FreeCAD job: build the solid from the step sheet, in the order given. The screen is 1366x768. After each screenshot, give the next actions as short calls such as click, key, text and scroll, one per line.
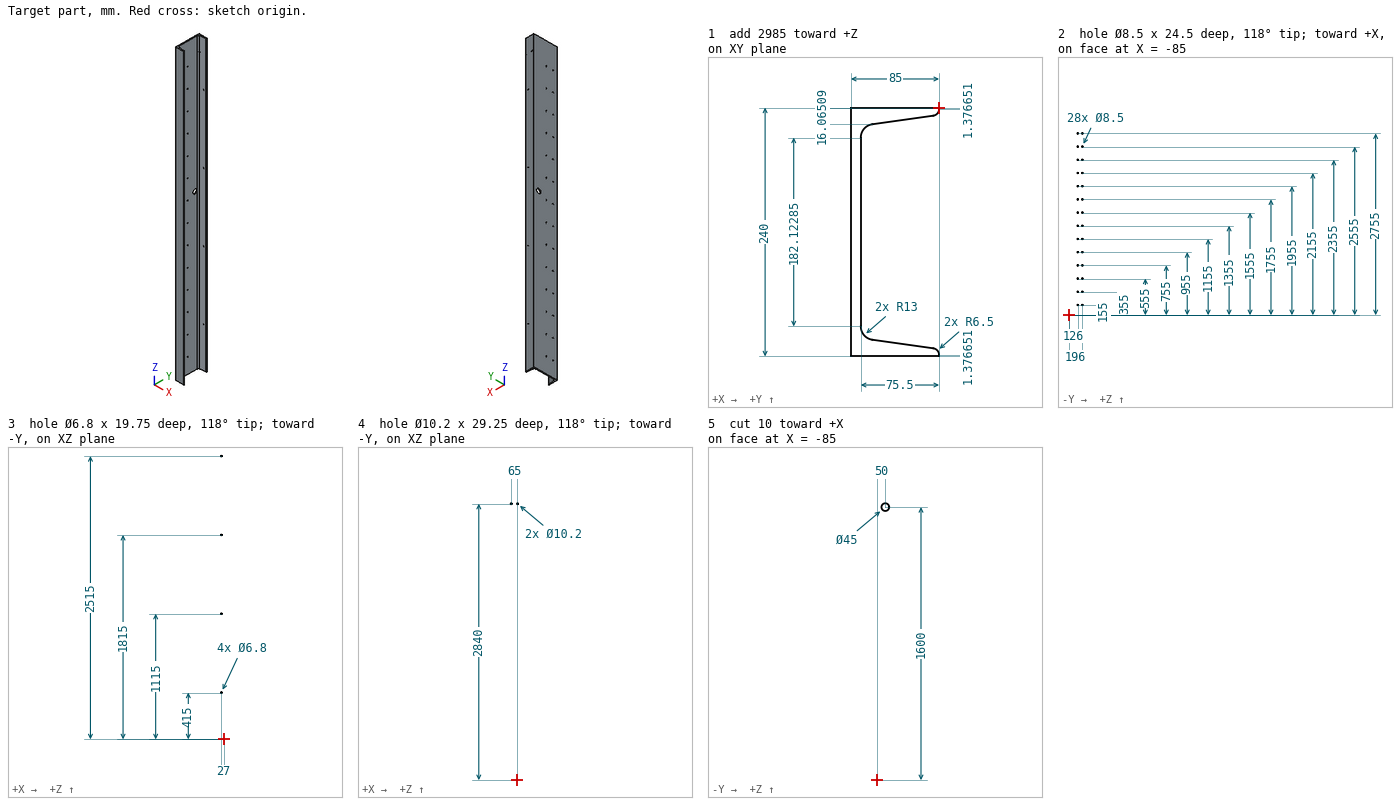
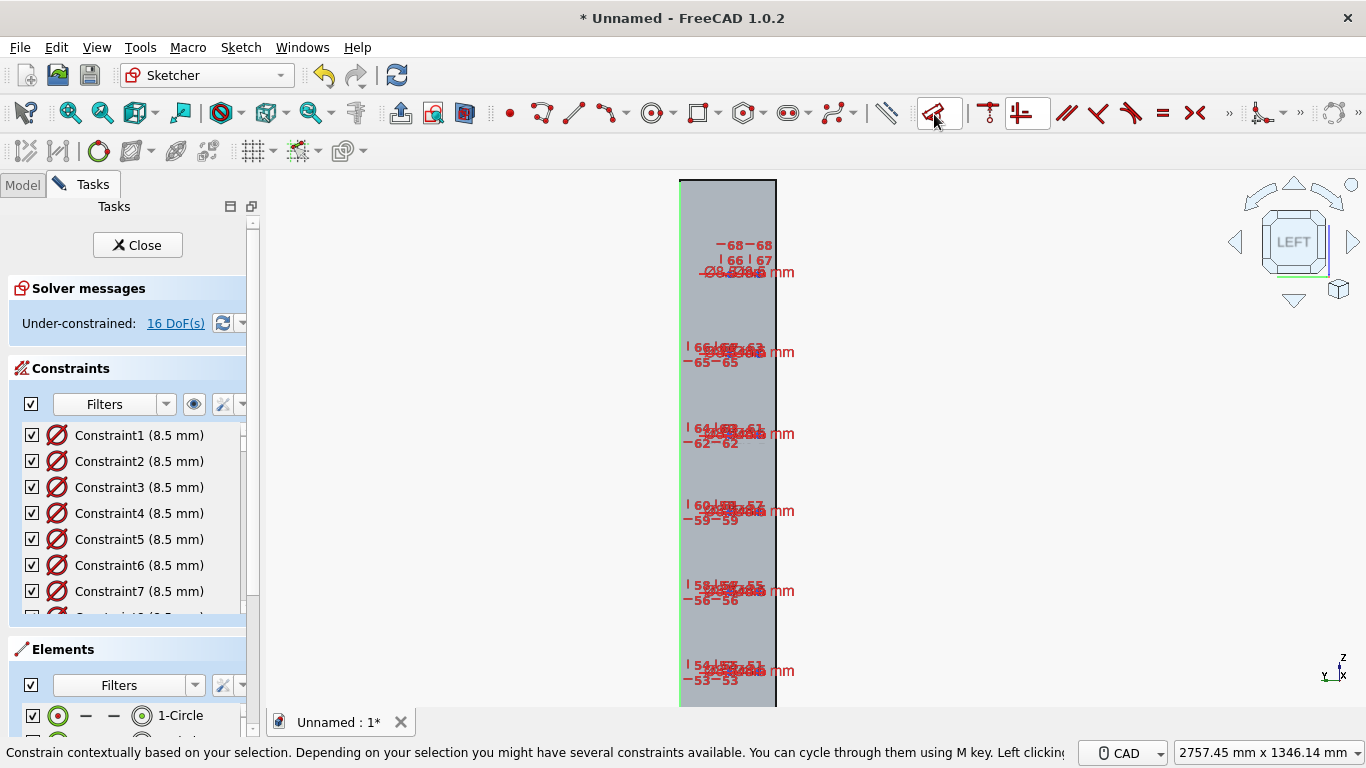
scroll(759, 274, down, 6)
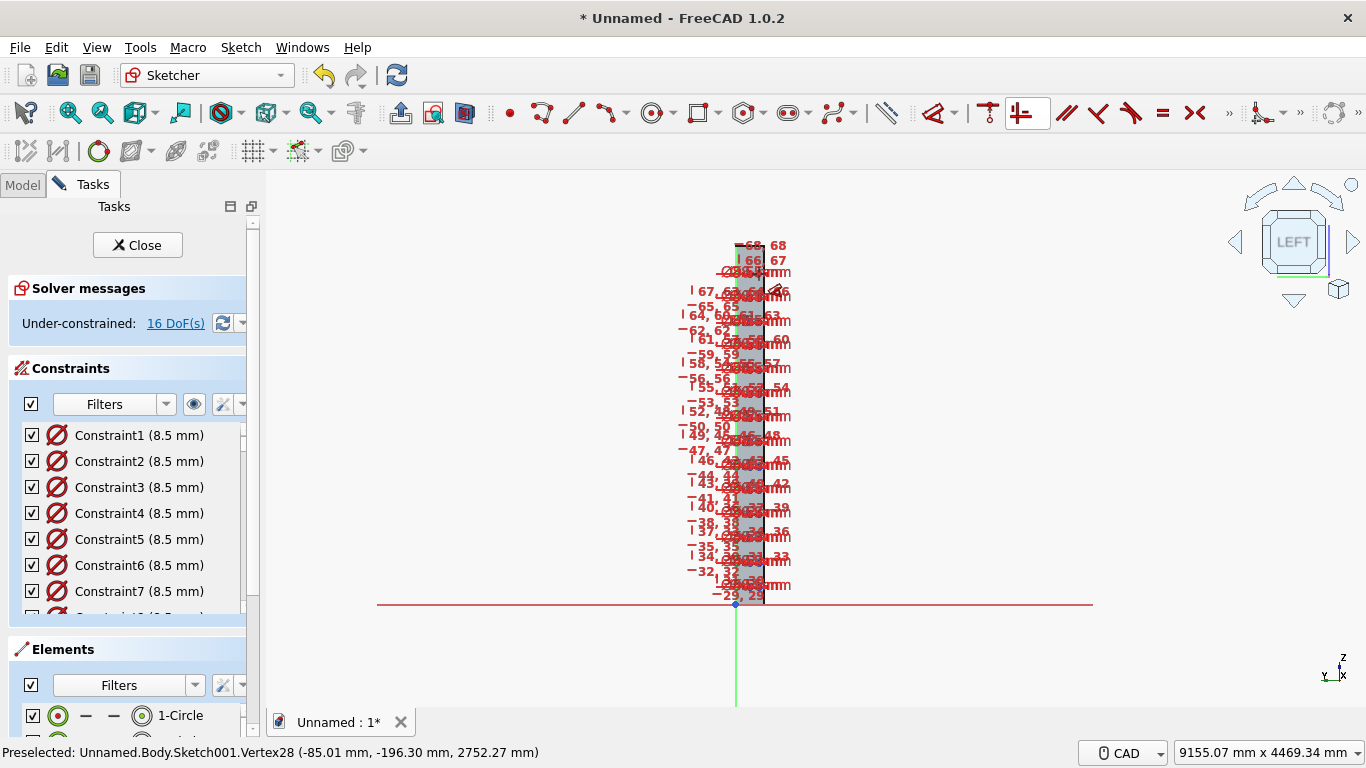
scroll(750, 587, up, 5)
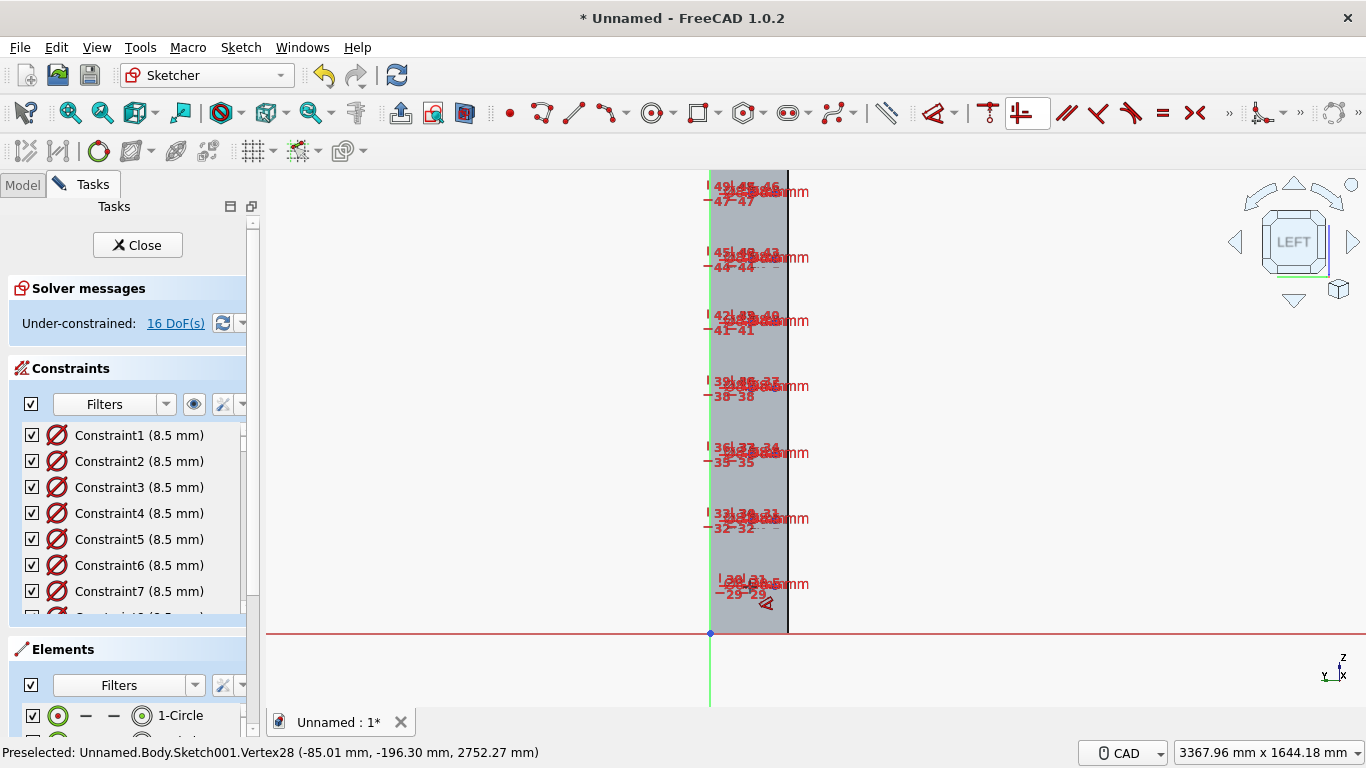
click(750, 586)
click(730, 668)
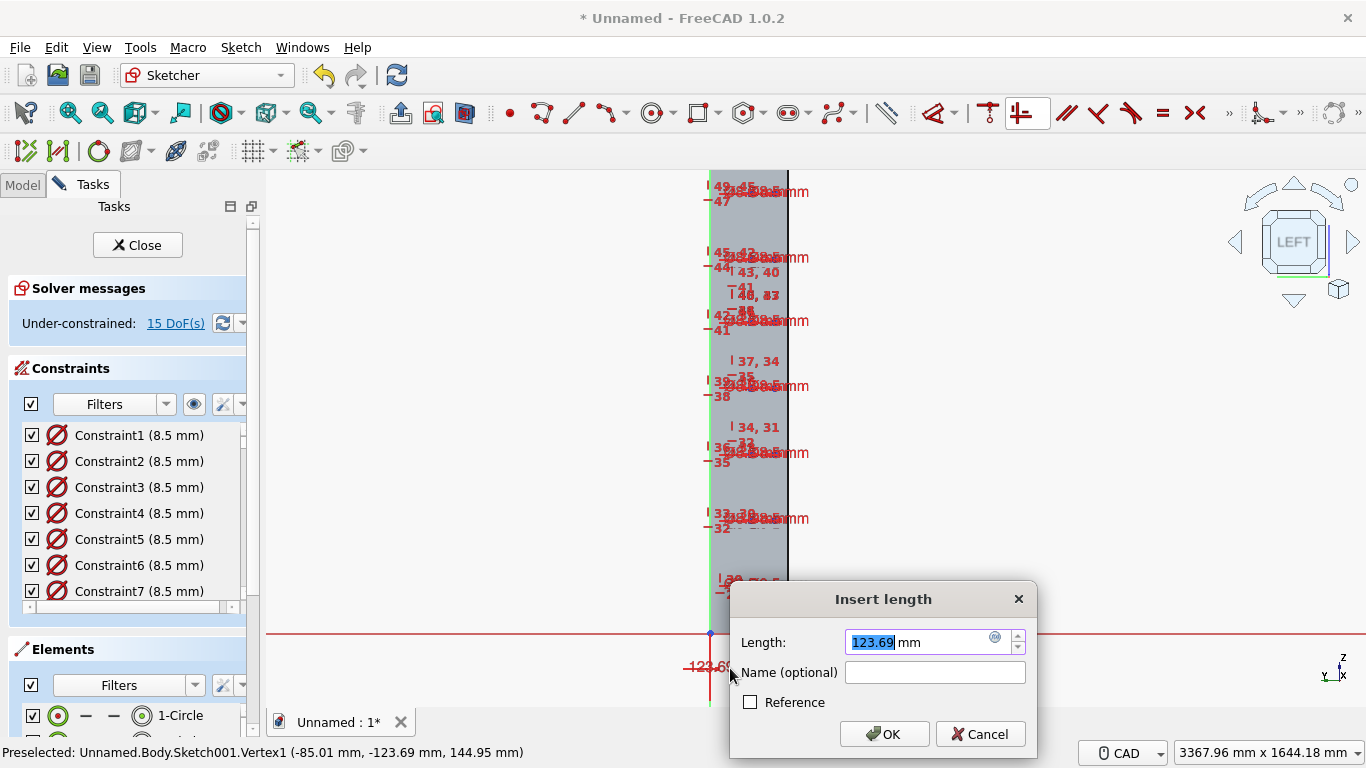
text(126)
key(Return)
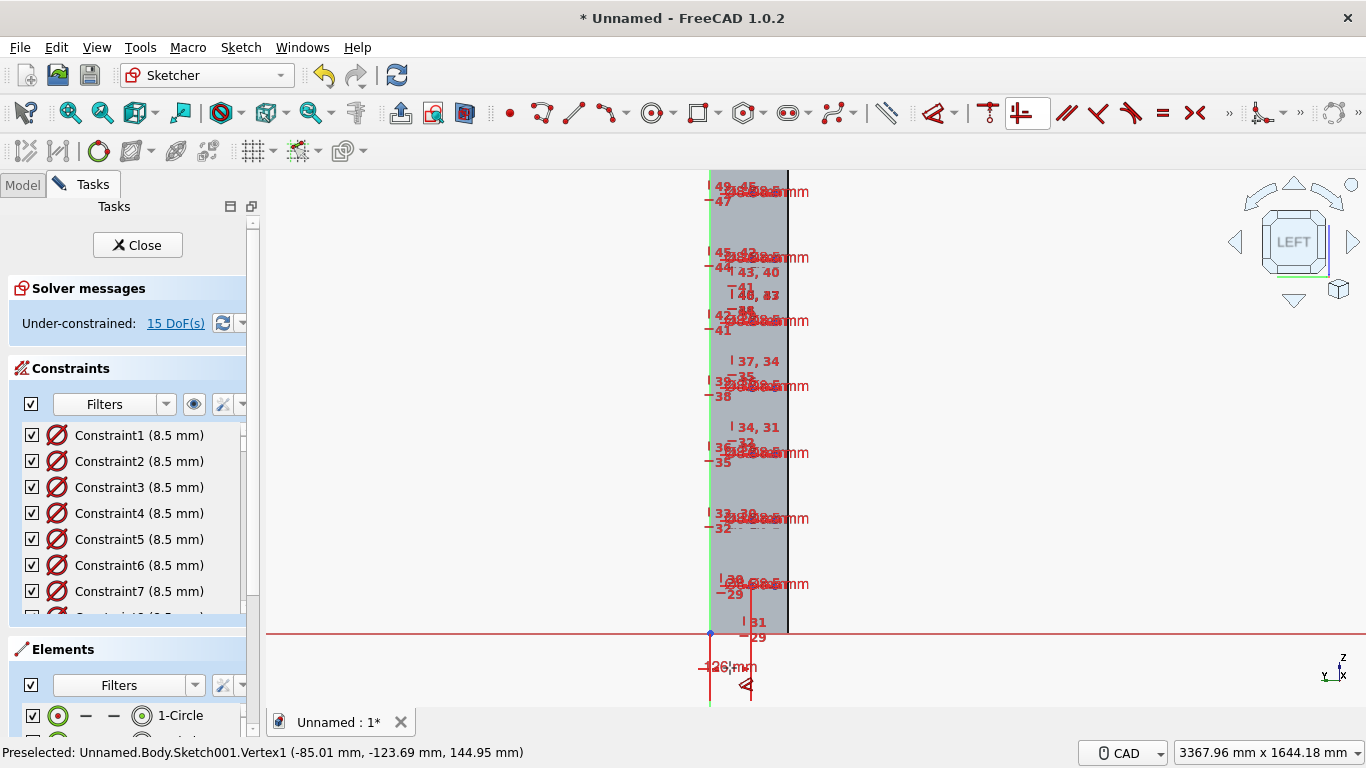
click(751, 586)
click(676, 610)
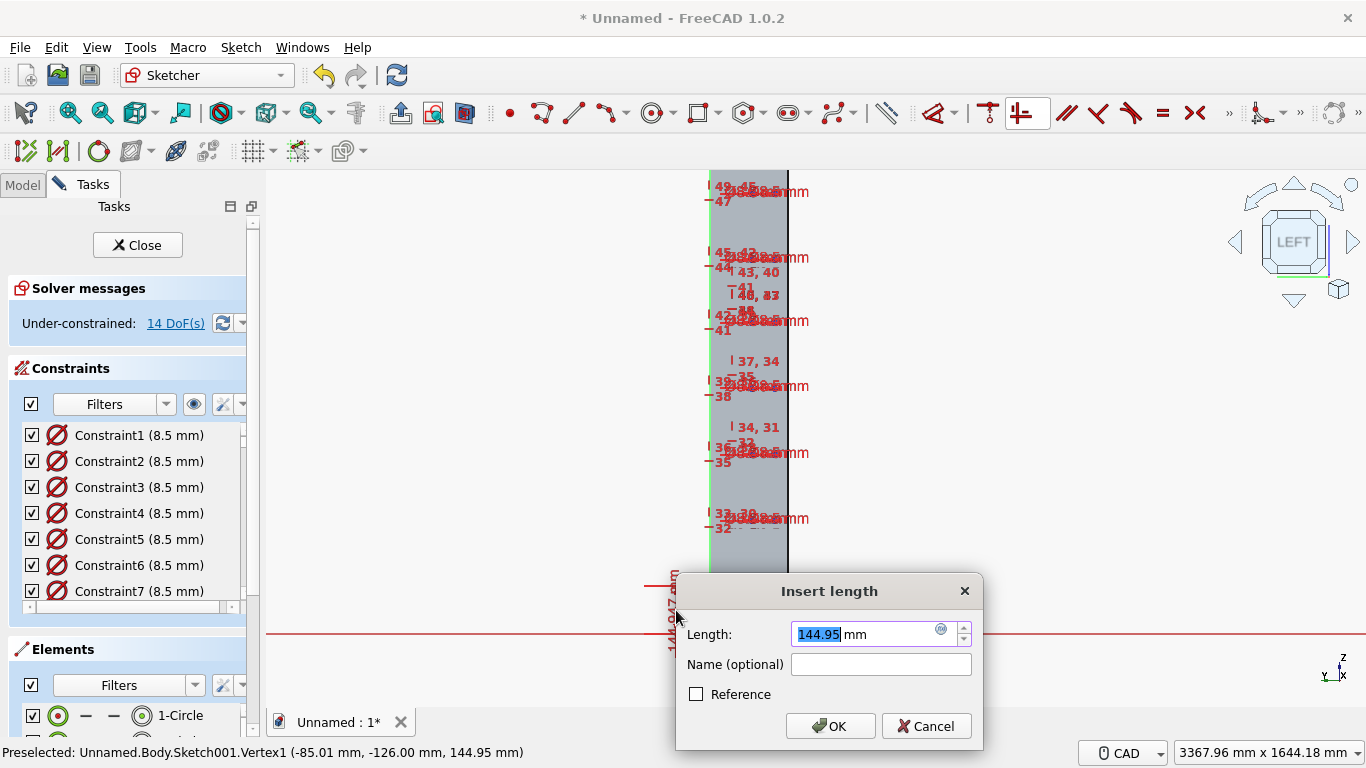
text(155)
key(Return)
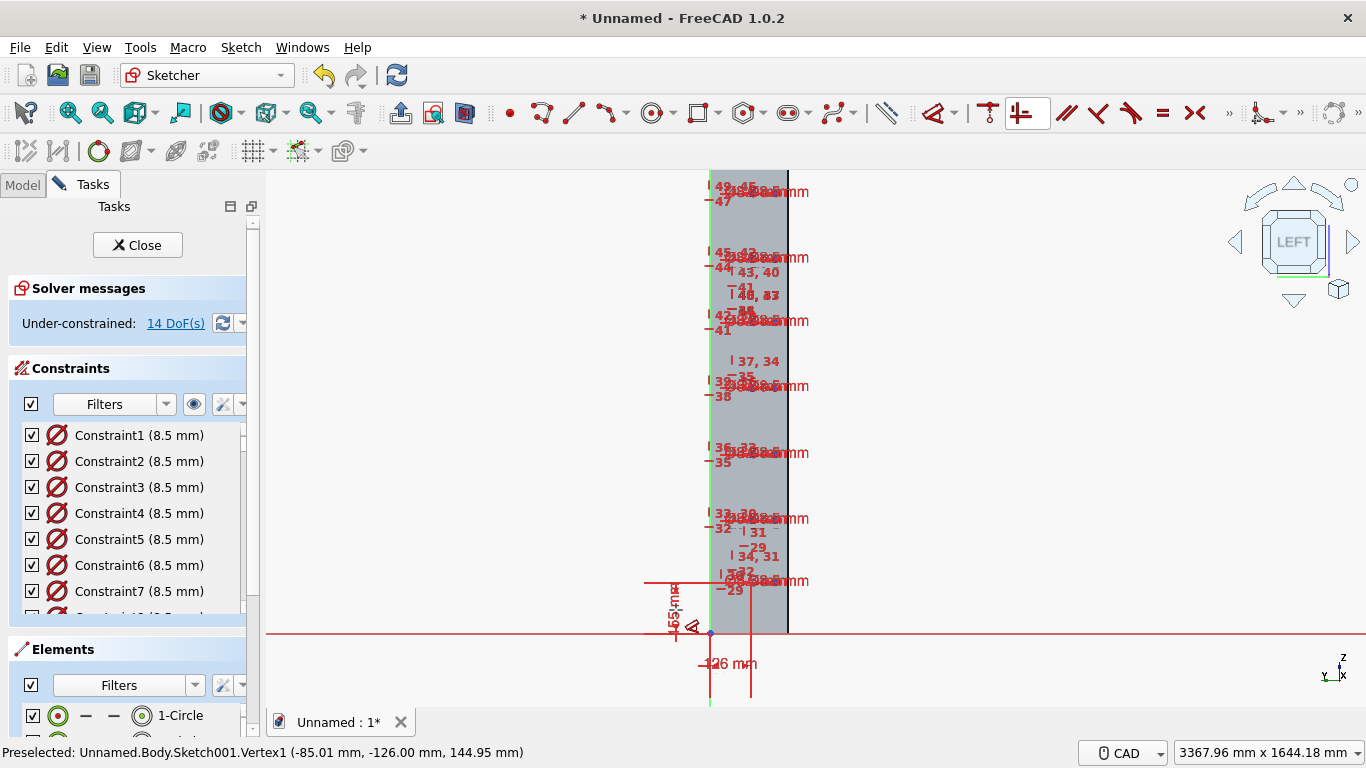
click(774, 583)
click(742, 549)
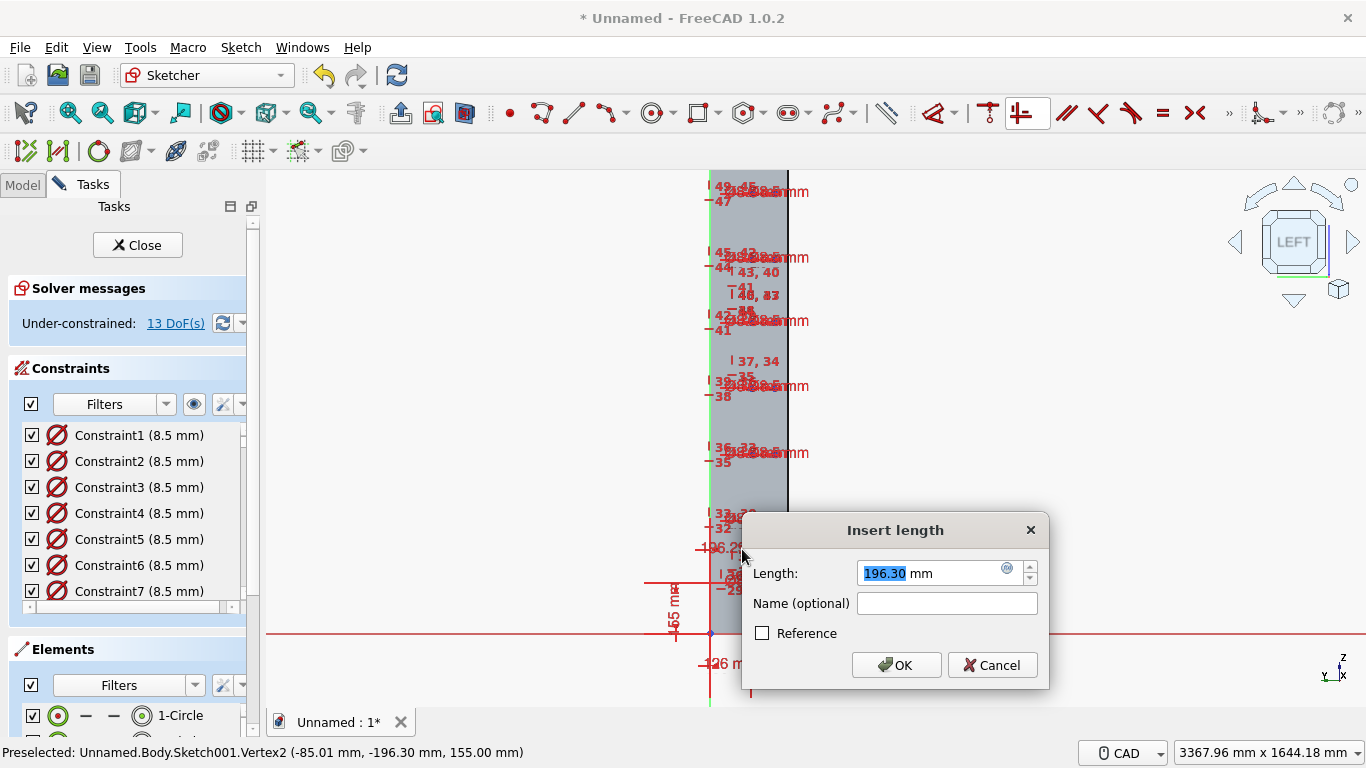
text(196)
key(Return)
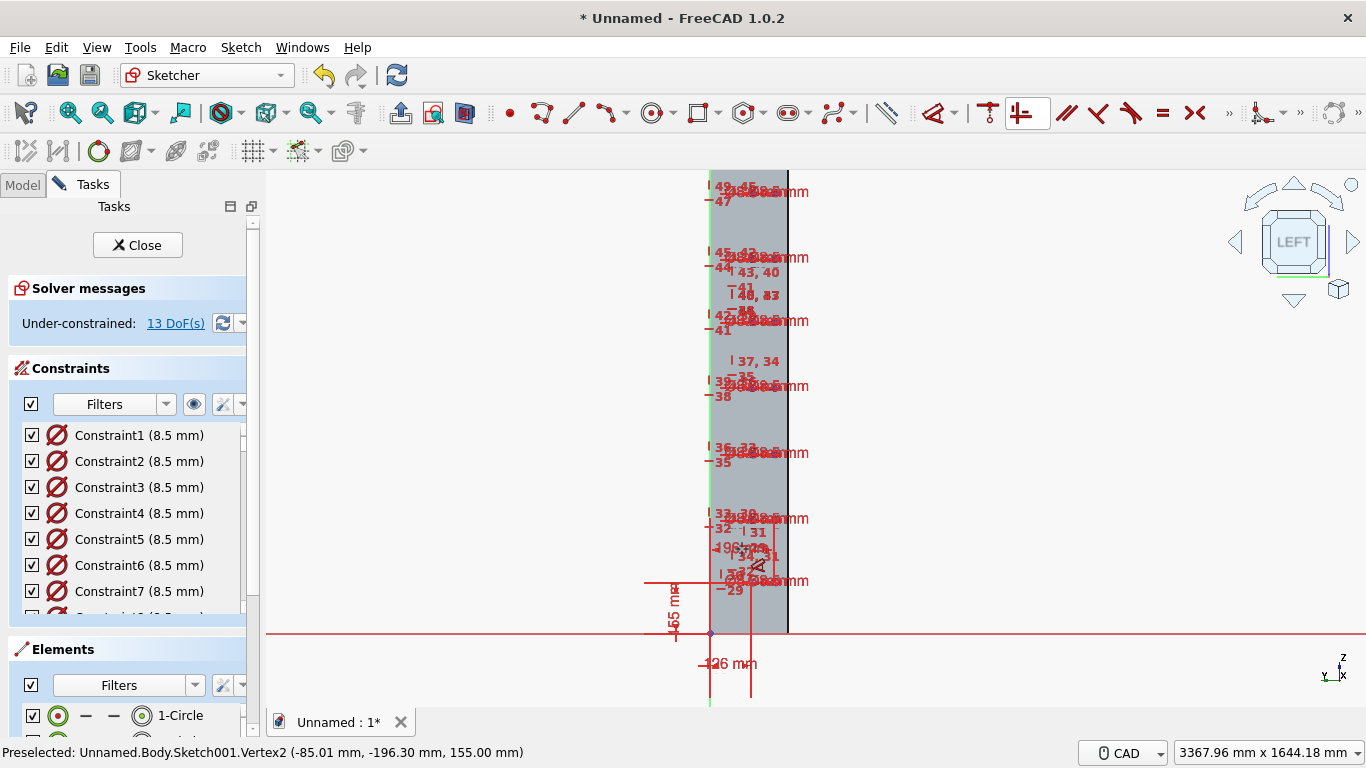
click(751, 521)
click(676, 577)